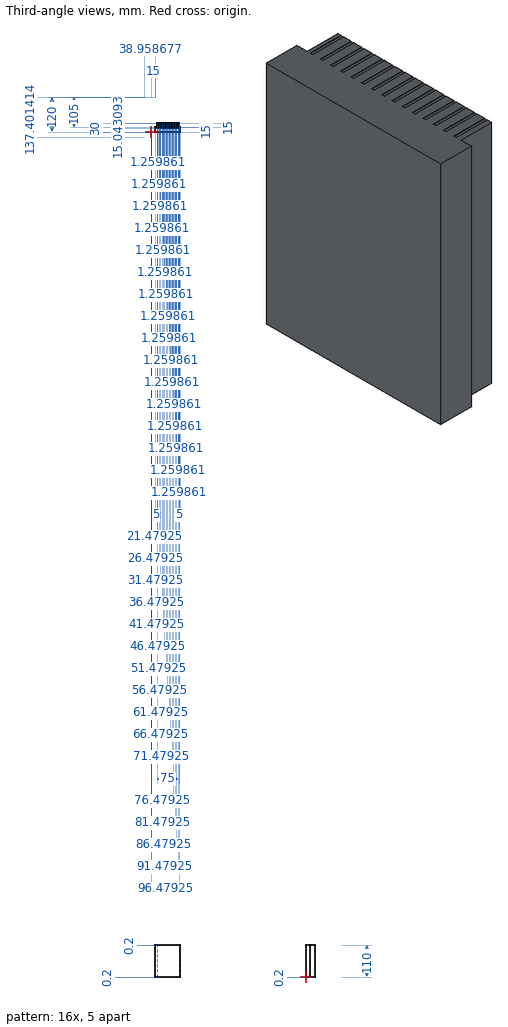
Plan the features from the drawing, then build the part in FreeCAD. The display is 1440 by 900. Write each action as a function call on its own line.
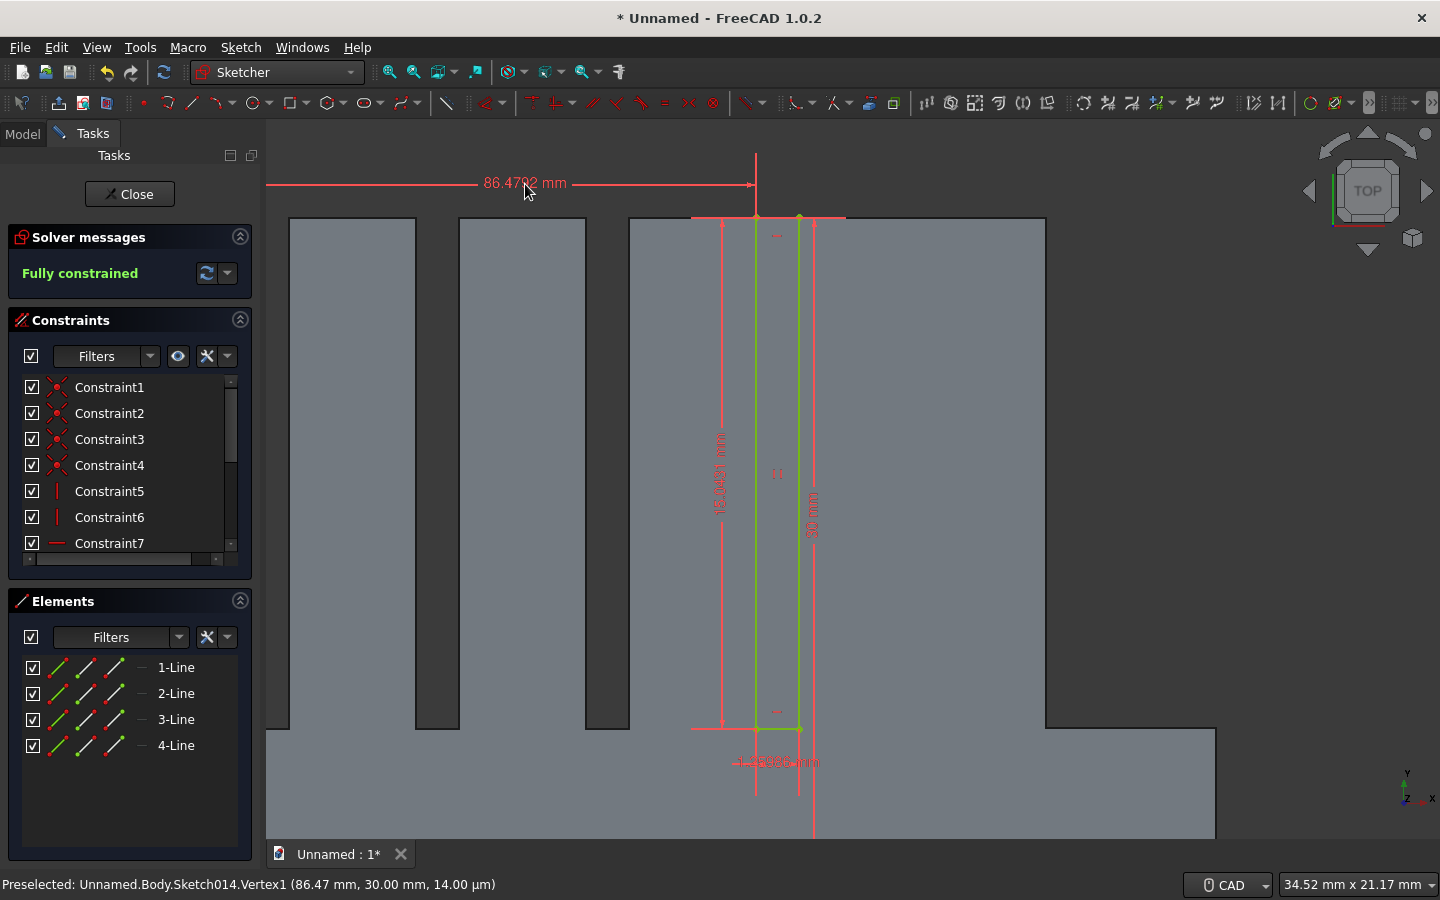
click(130, 194)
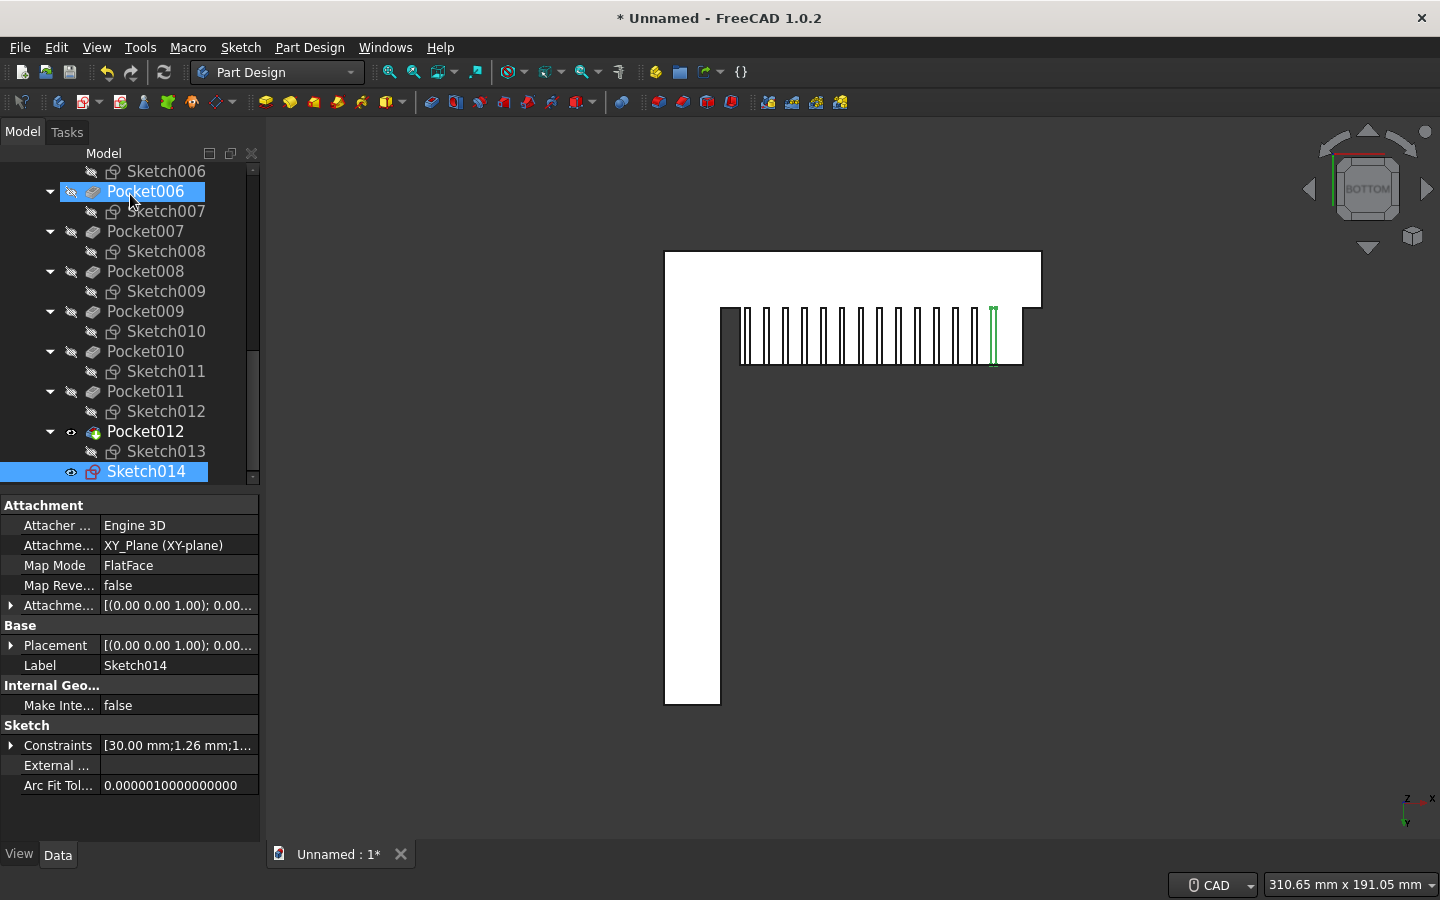
click(432, 102)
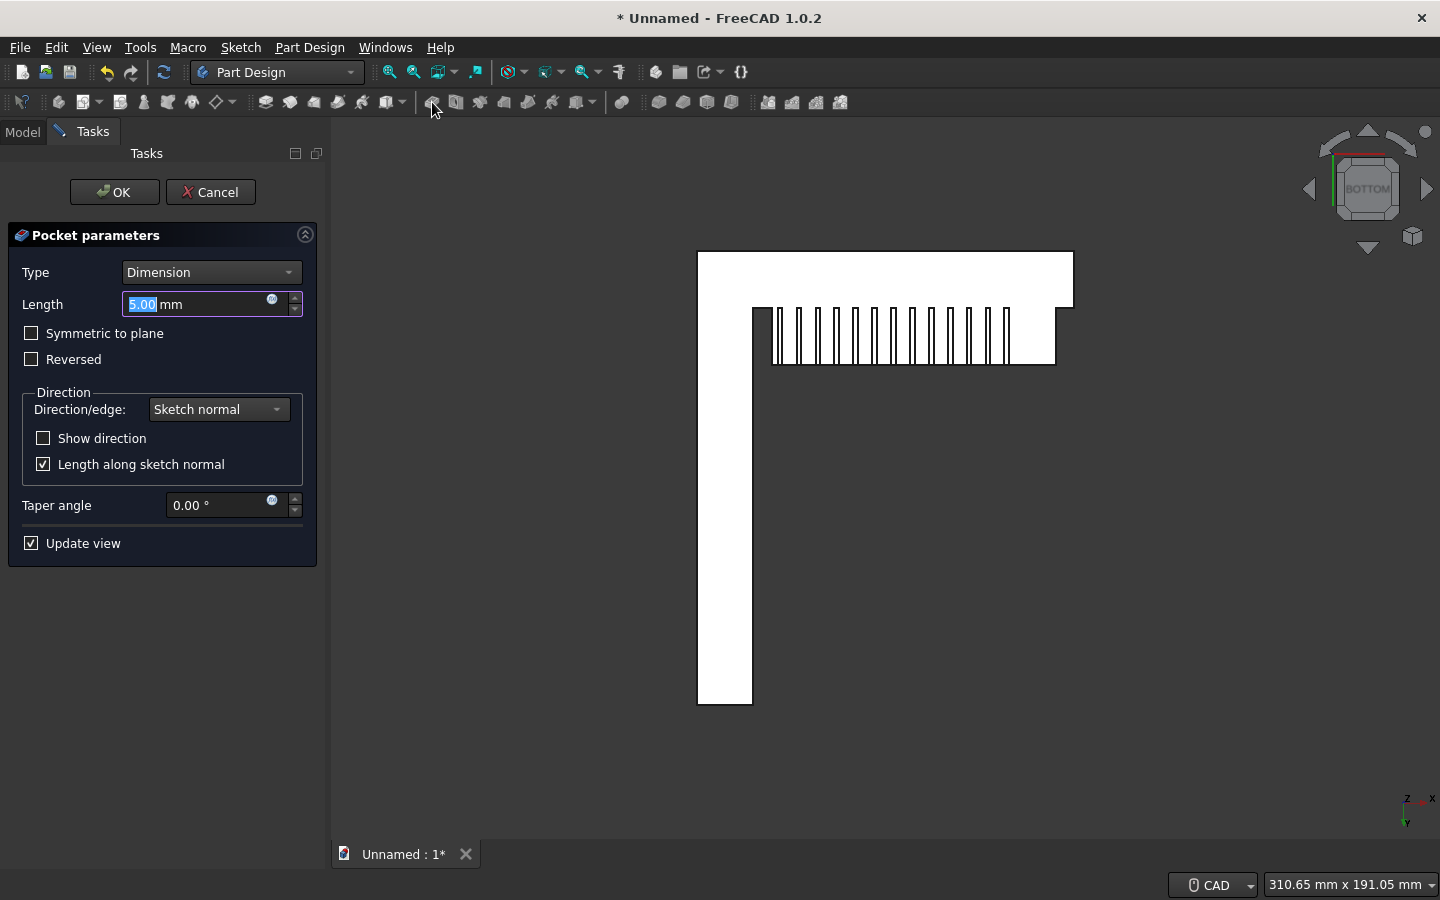
text(0.2)
key(Tab)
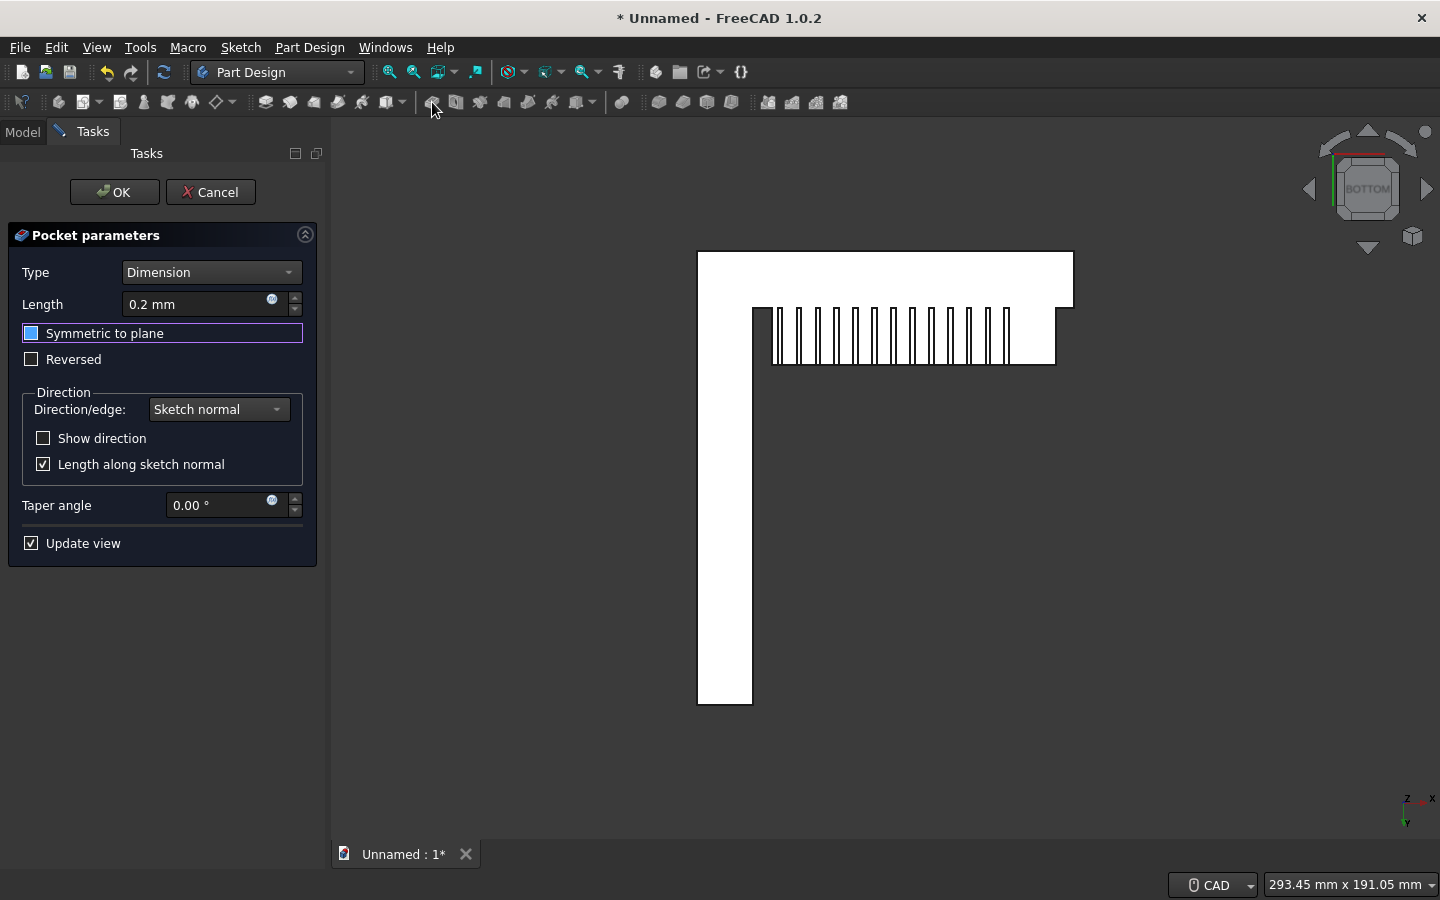
click(30, 359)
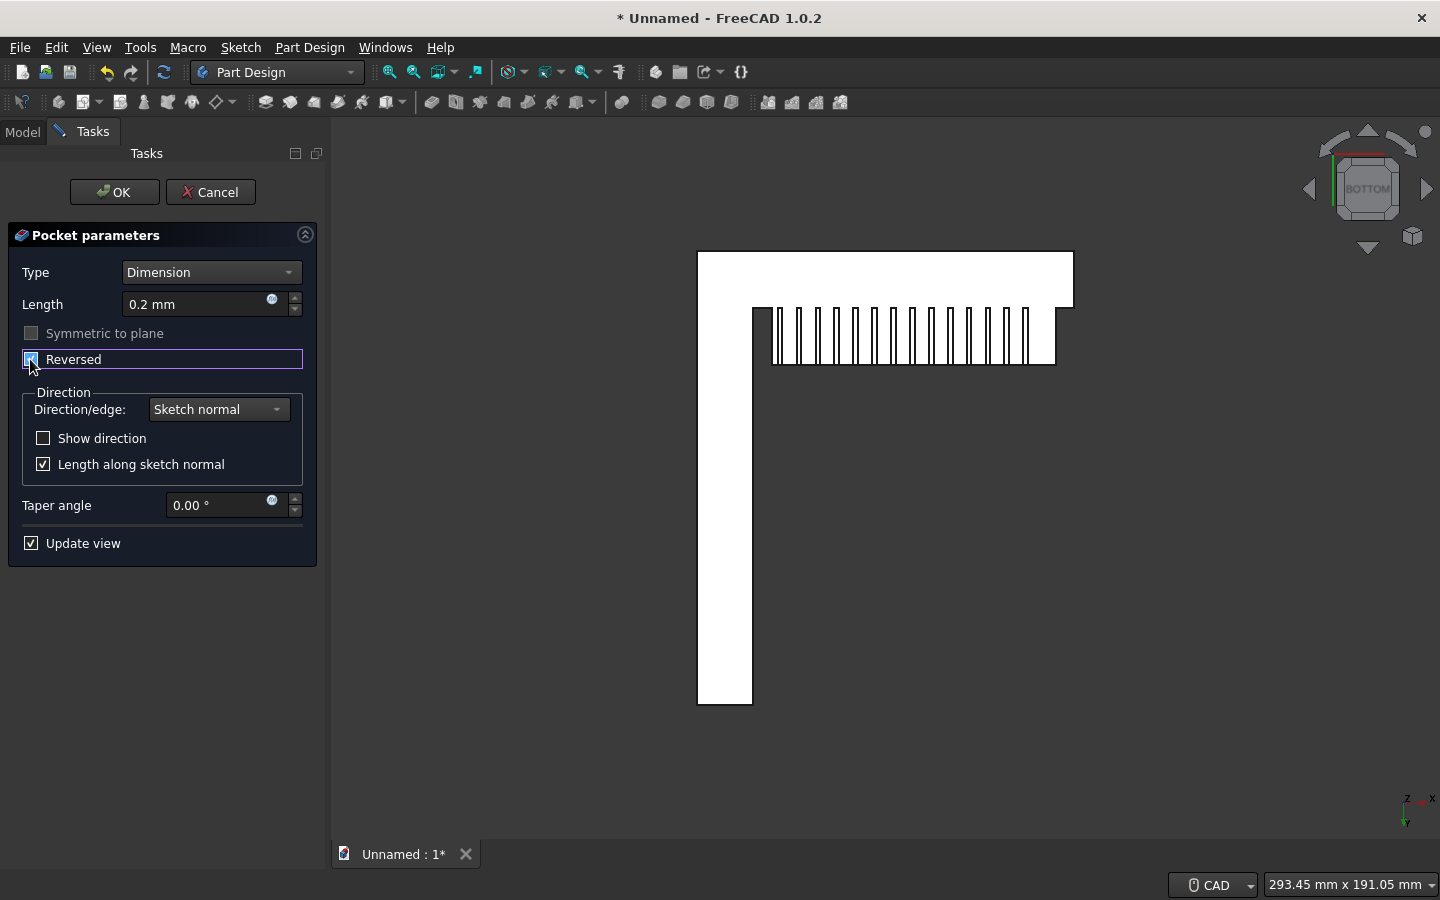
click(115, 192)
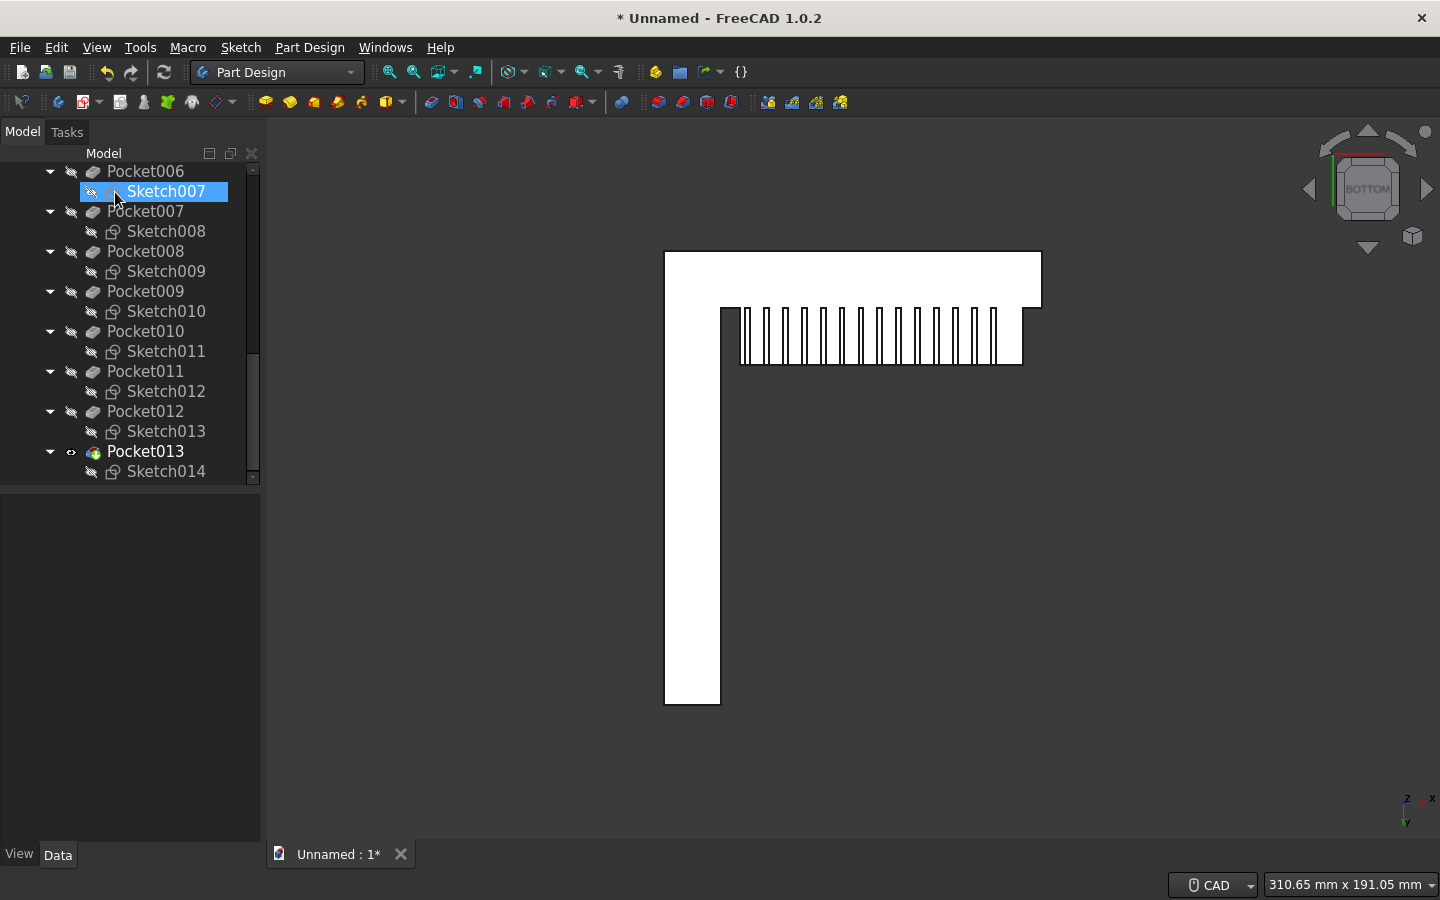
click(84, 102)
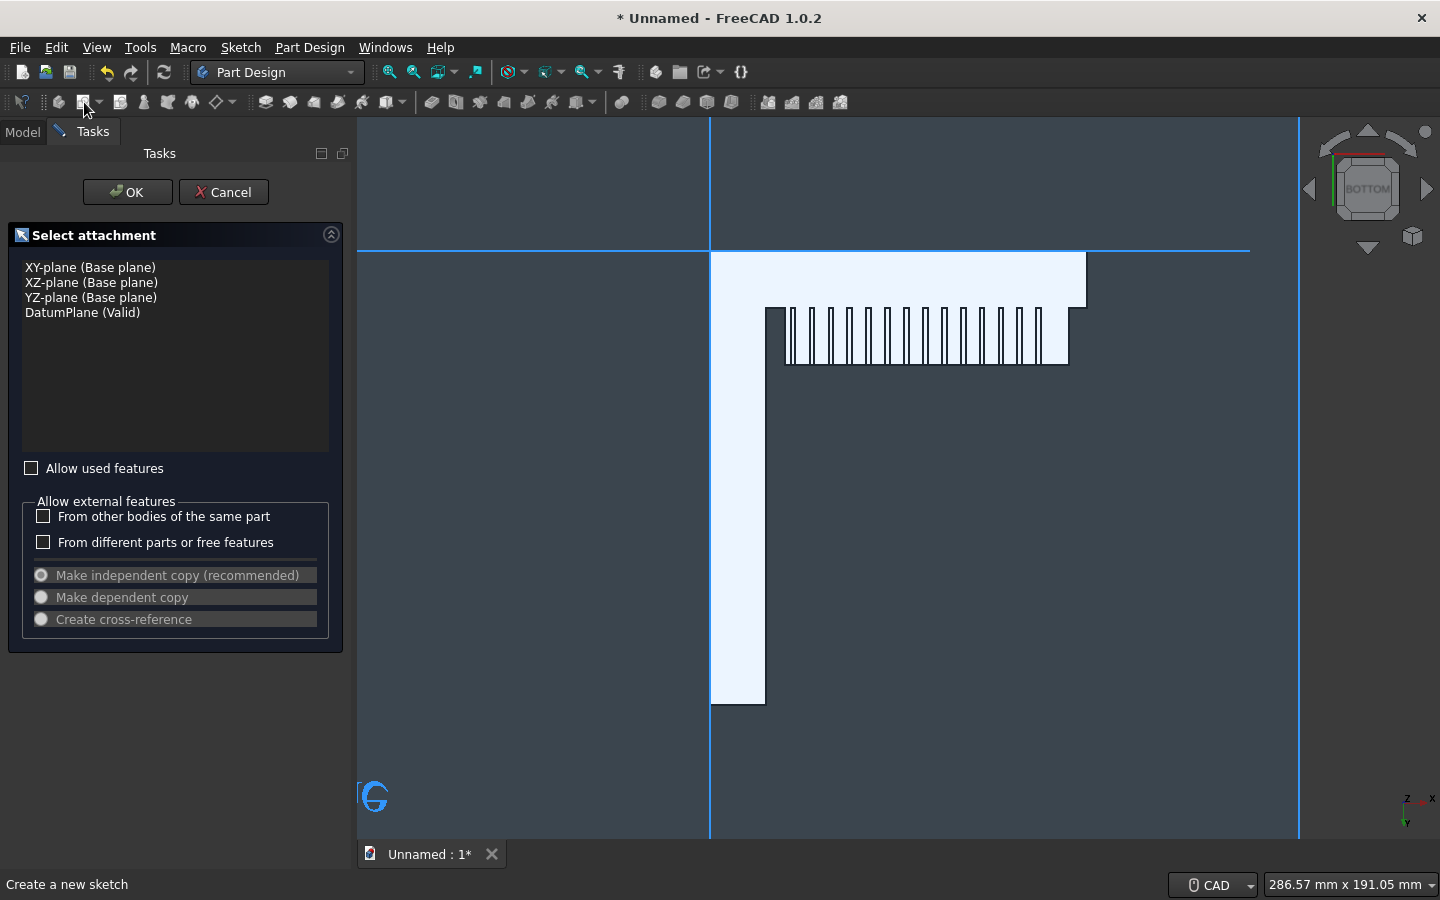
click(82, 268)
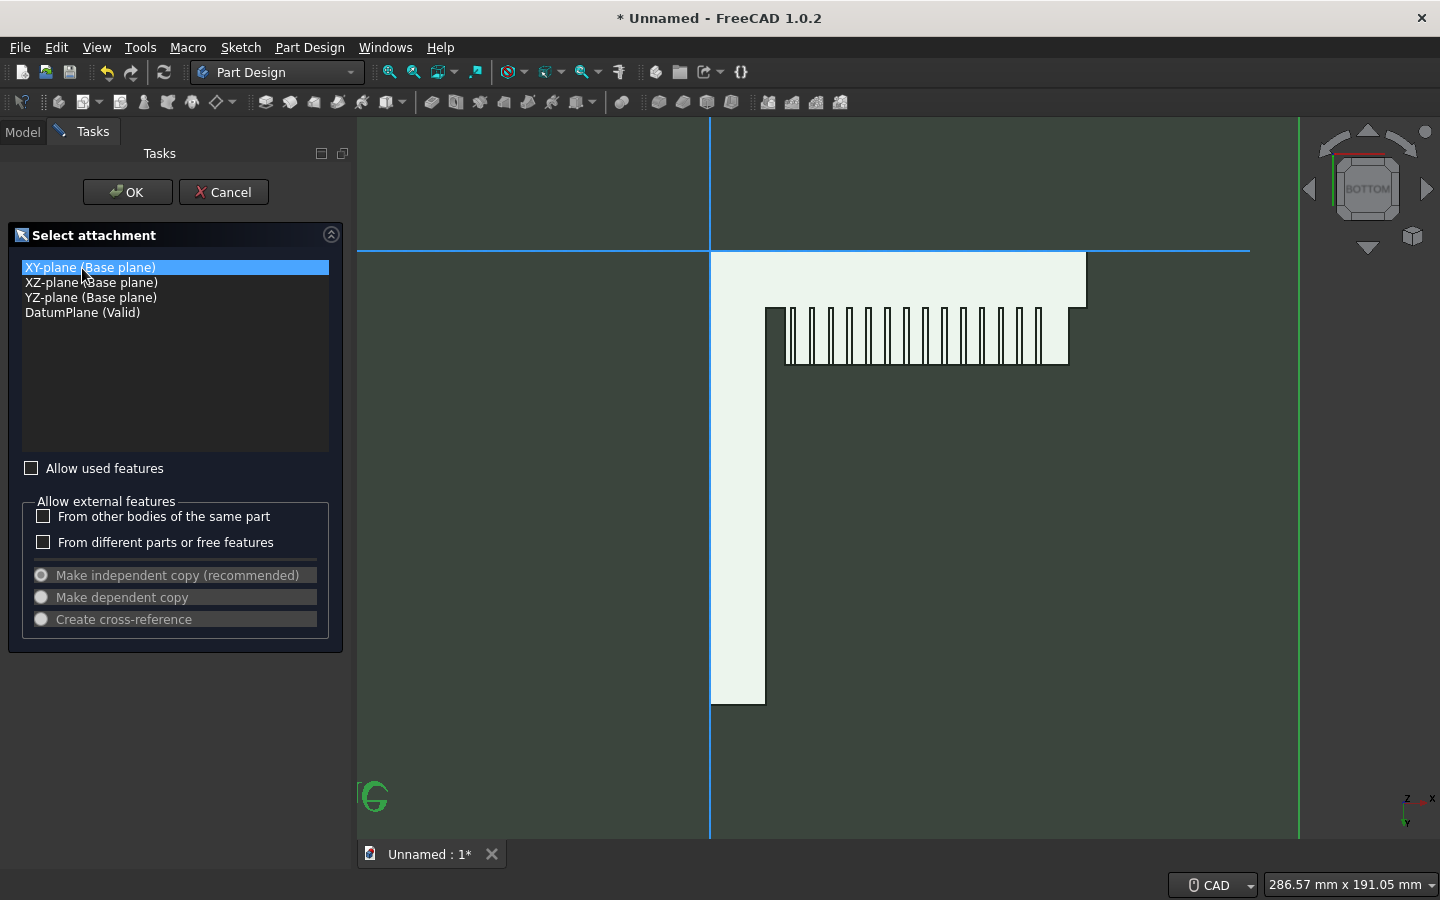
click(128, 192)